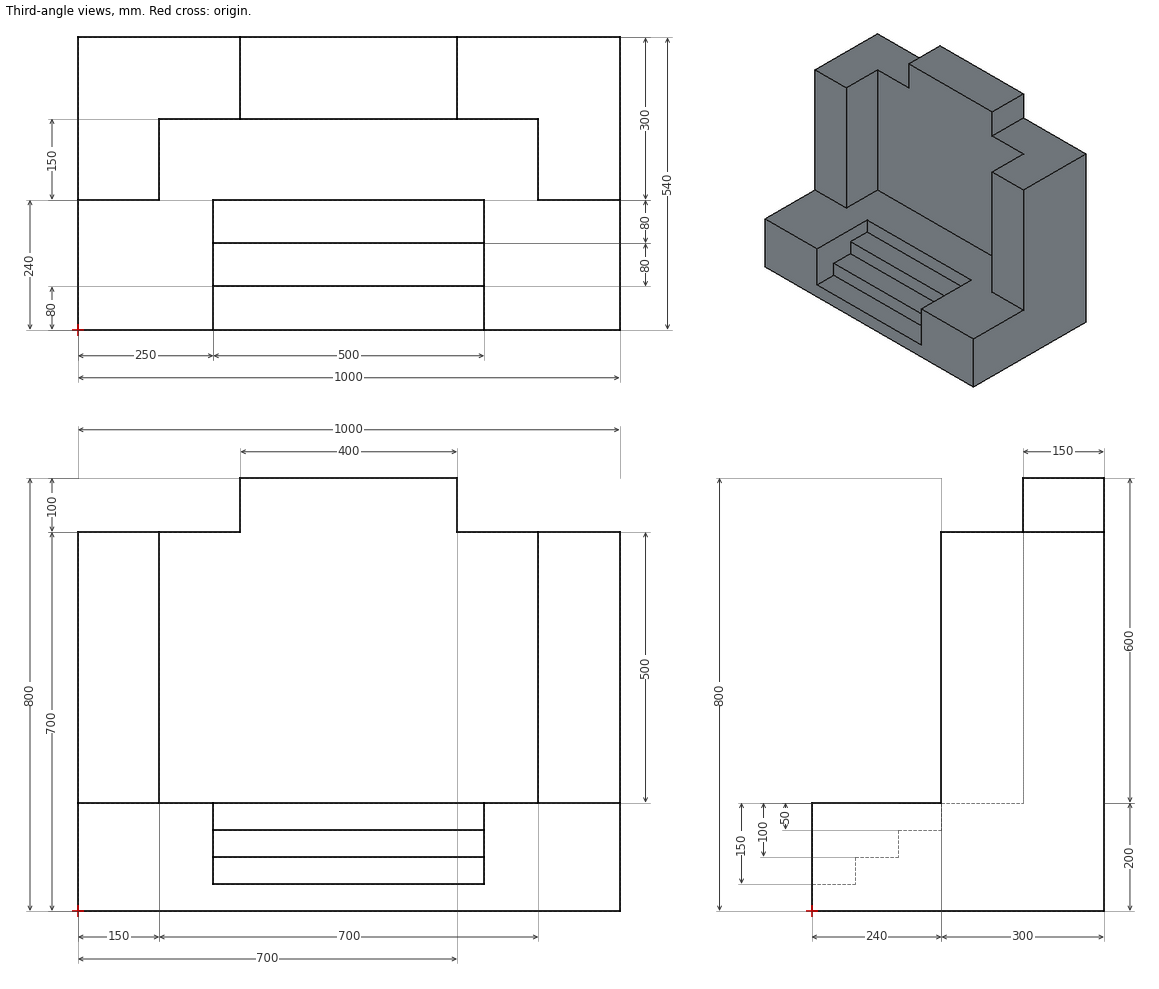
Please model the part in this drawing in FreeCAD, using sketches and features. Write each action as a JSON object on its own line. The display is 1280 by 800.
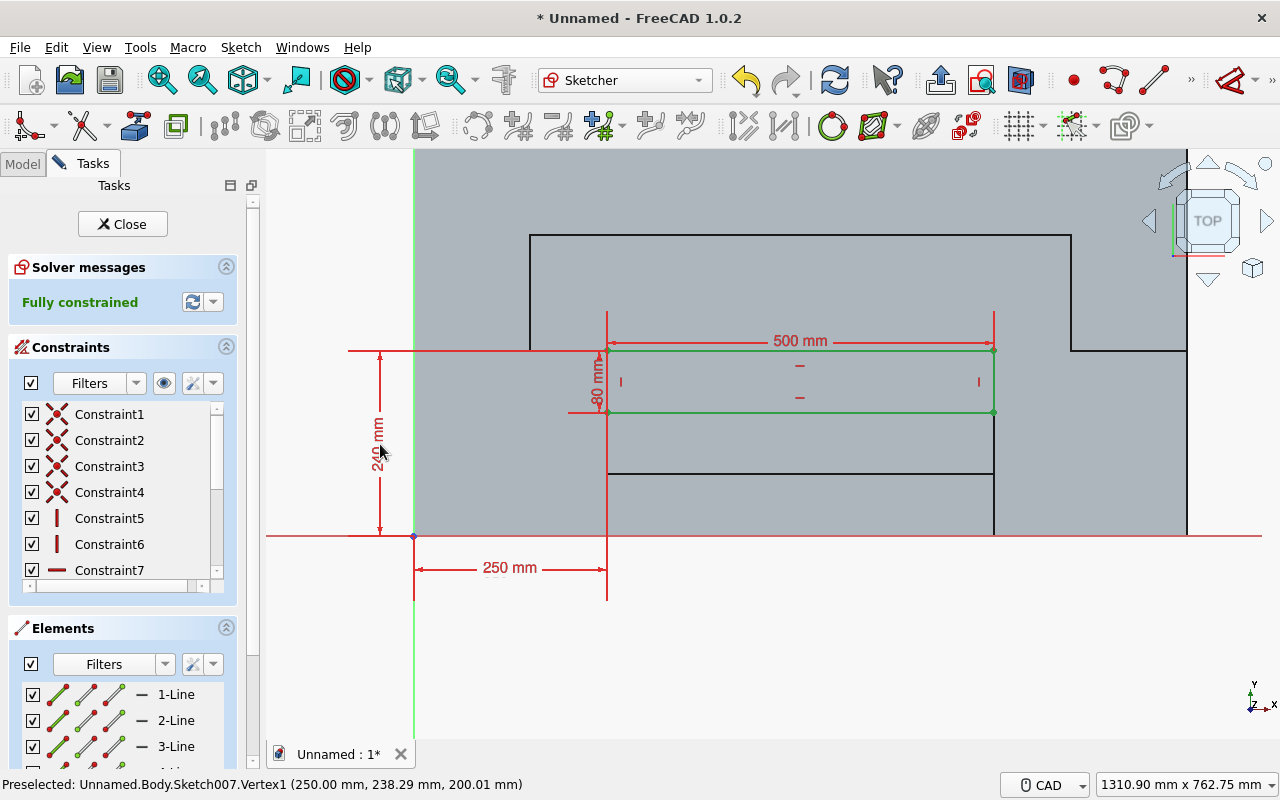
{"action": "left_click", "coordinate": [123, 224]}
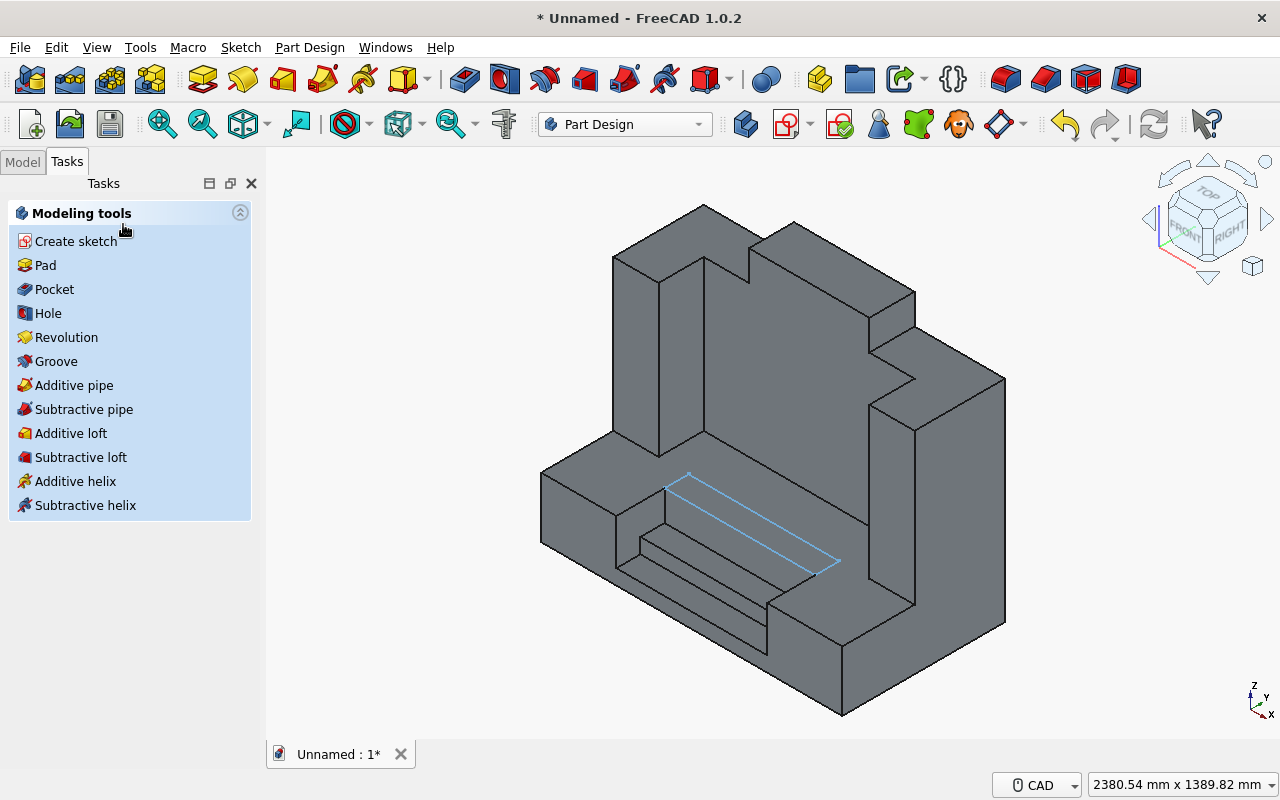
{"action": "left_click", "coordinate": [466, 80]}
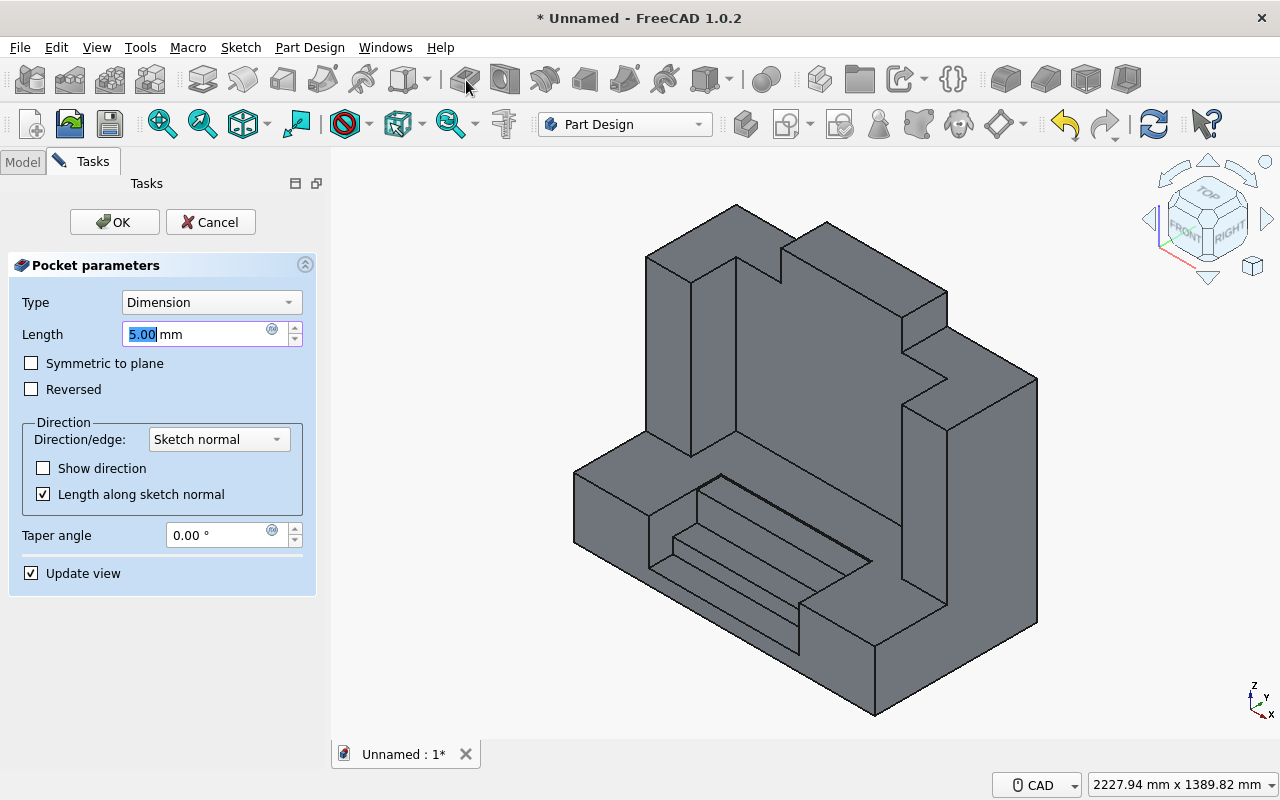
{"action": "type", "text": "50"}
{"action": "key", "text": "Tab"}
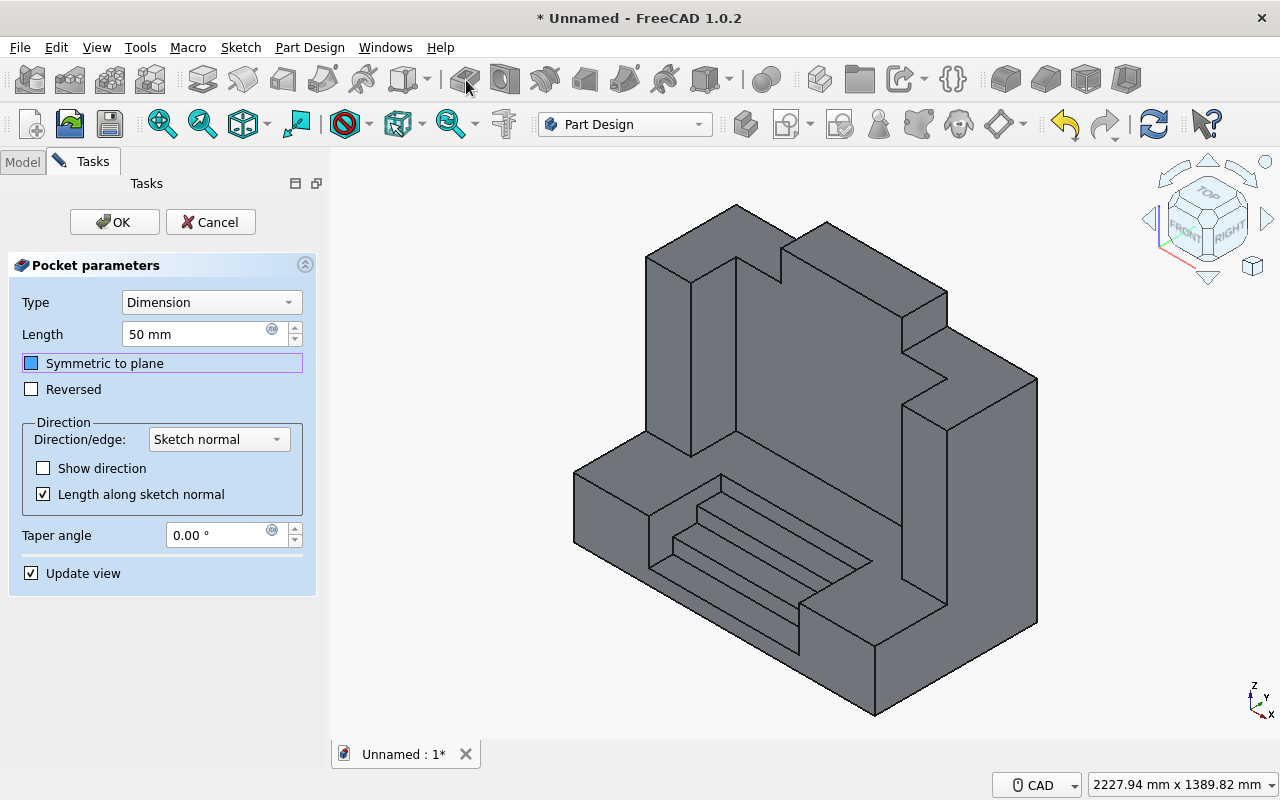
{"action": "left_click", "coordinate": [115, 222]}